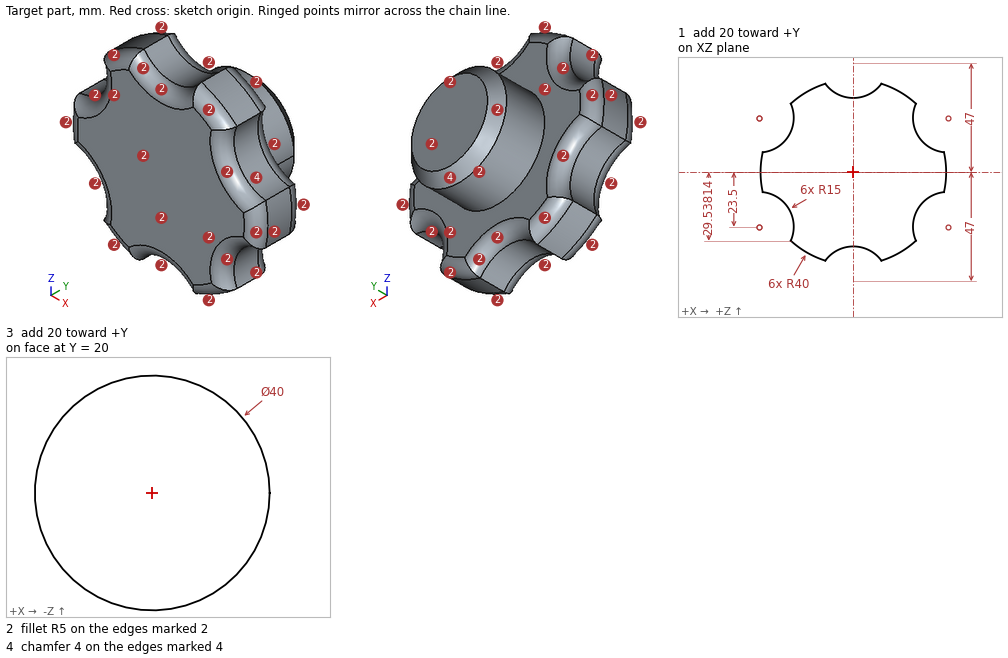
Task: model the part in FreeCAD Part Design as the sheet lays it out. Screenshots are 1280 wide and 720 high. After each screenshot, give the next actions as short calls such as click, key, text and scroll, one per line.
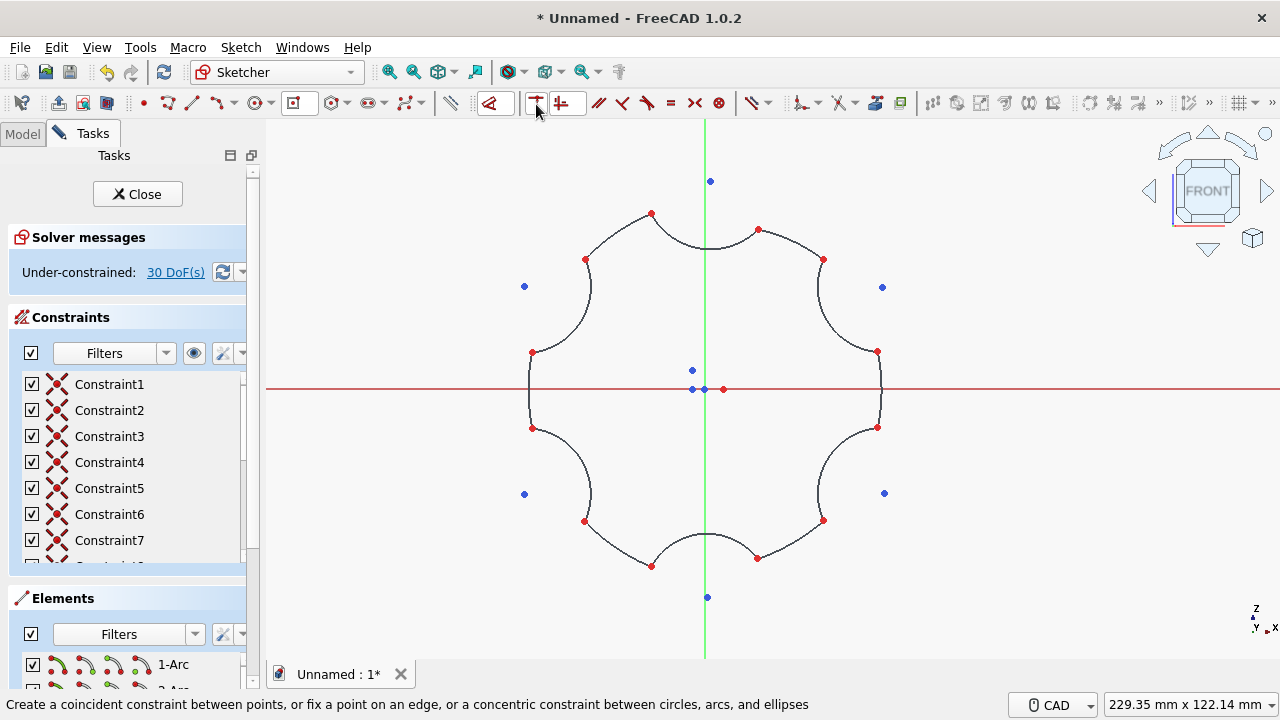
click(603, 538)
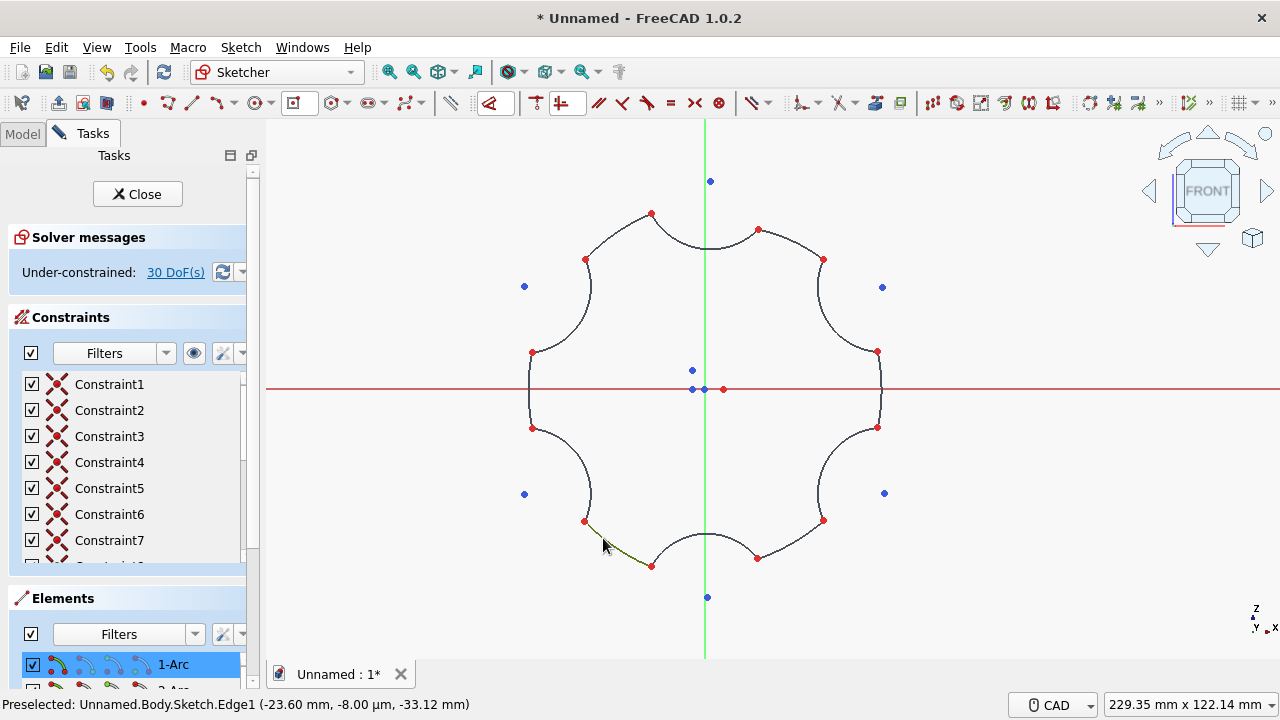
click(881, 405)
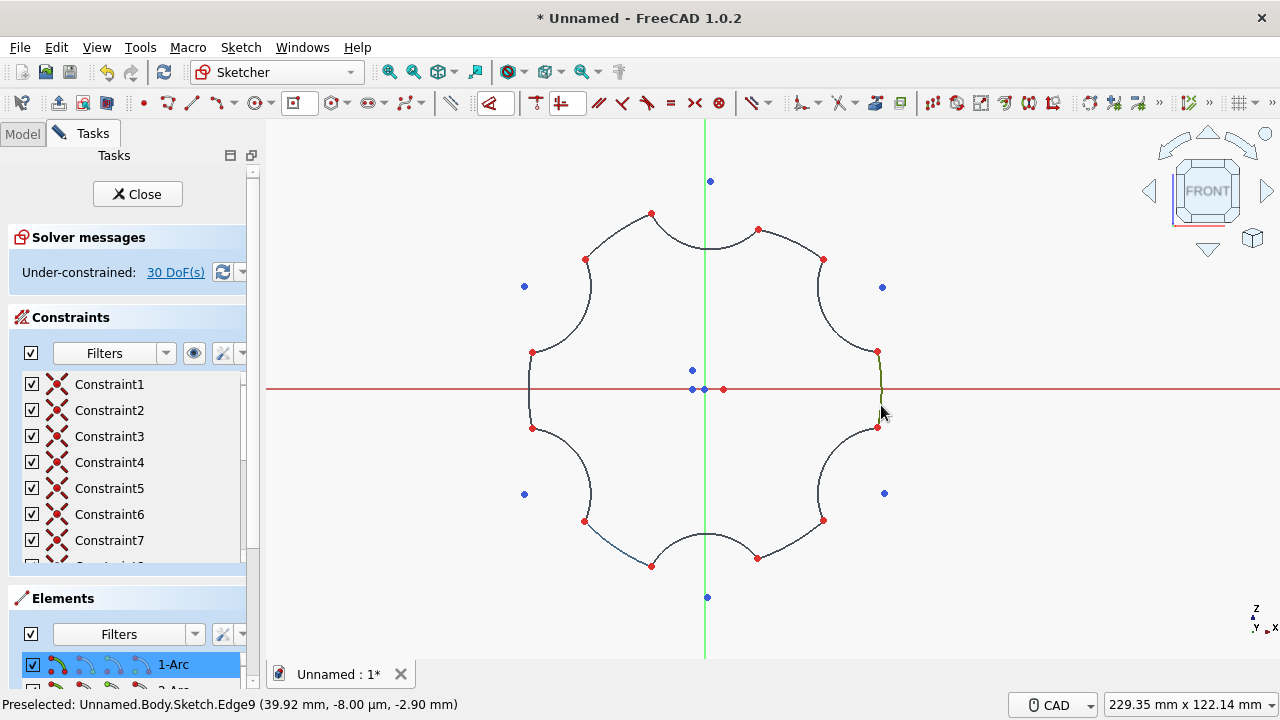
click(536, 104)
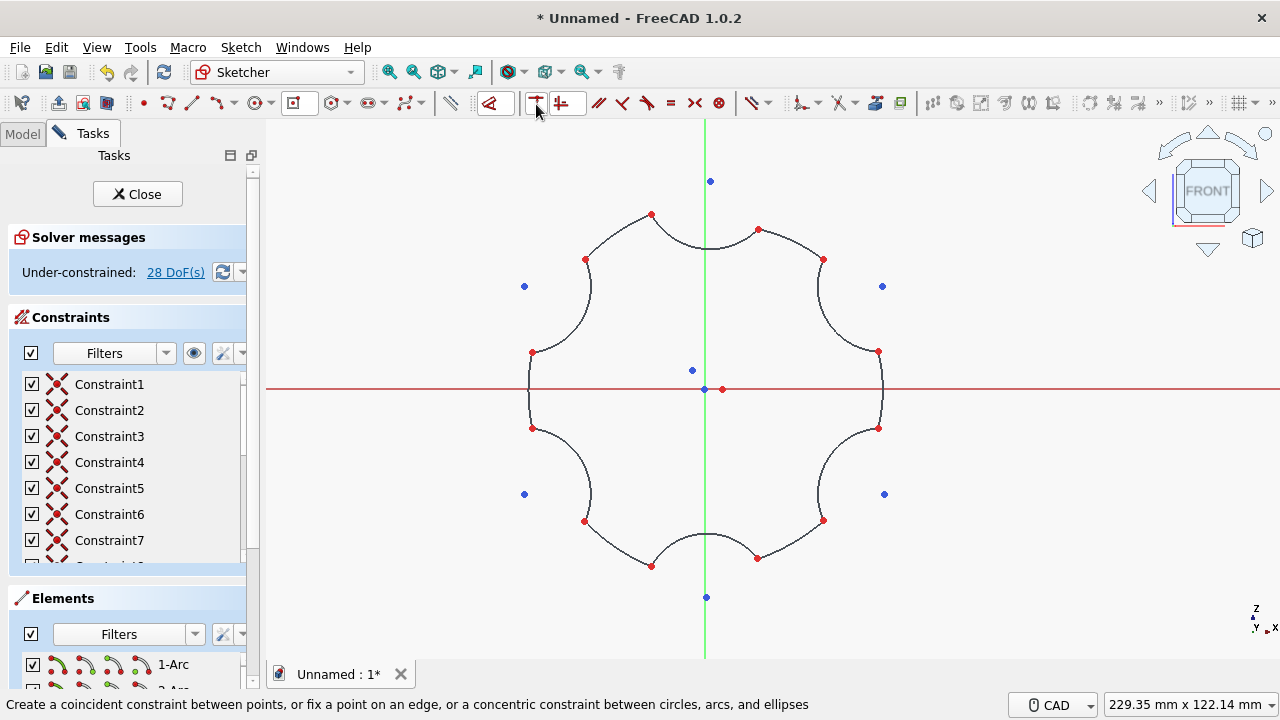
click(603, 538)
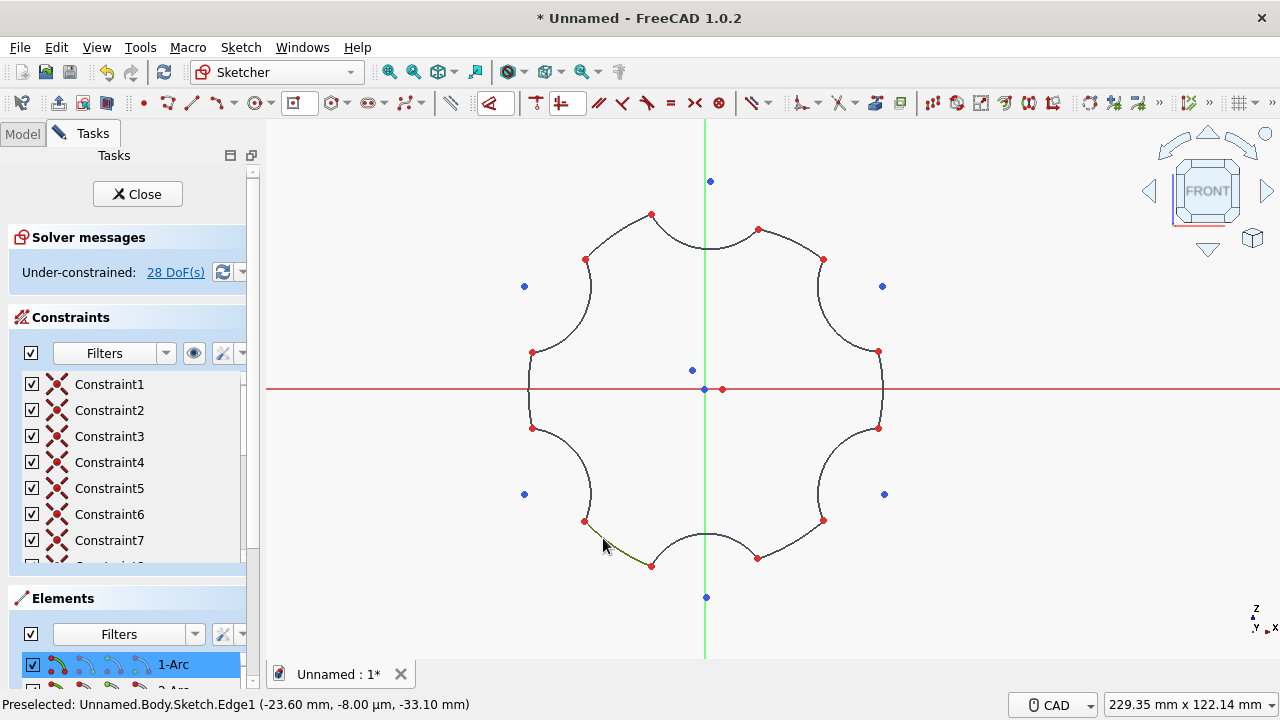
click(779, 550)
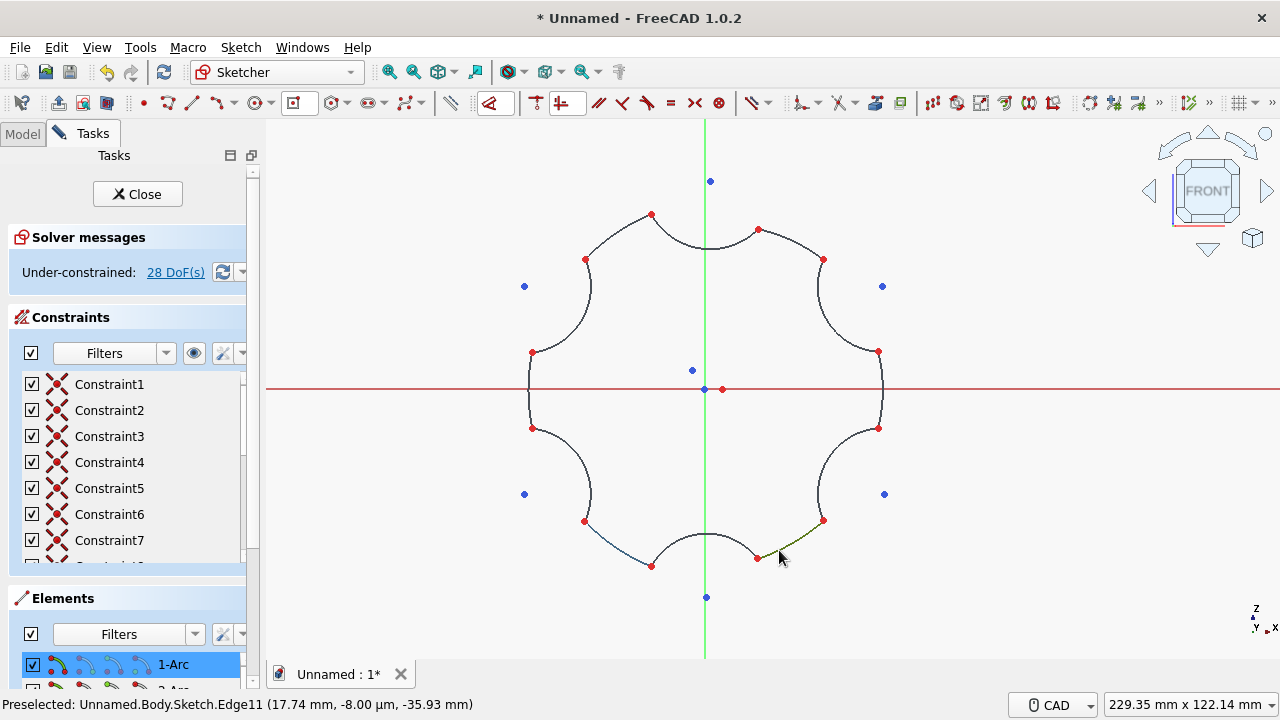
click(536, 104)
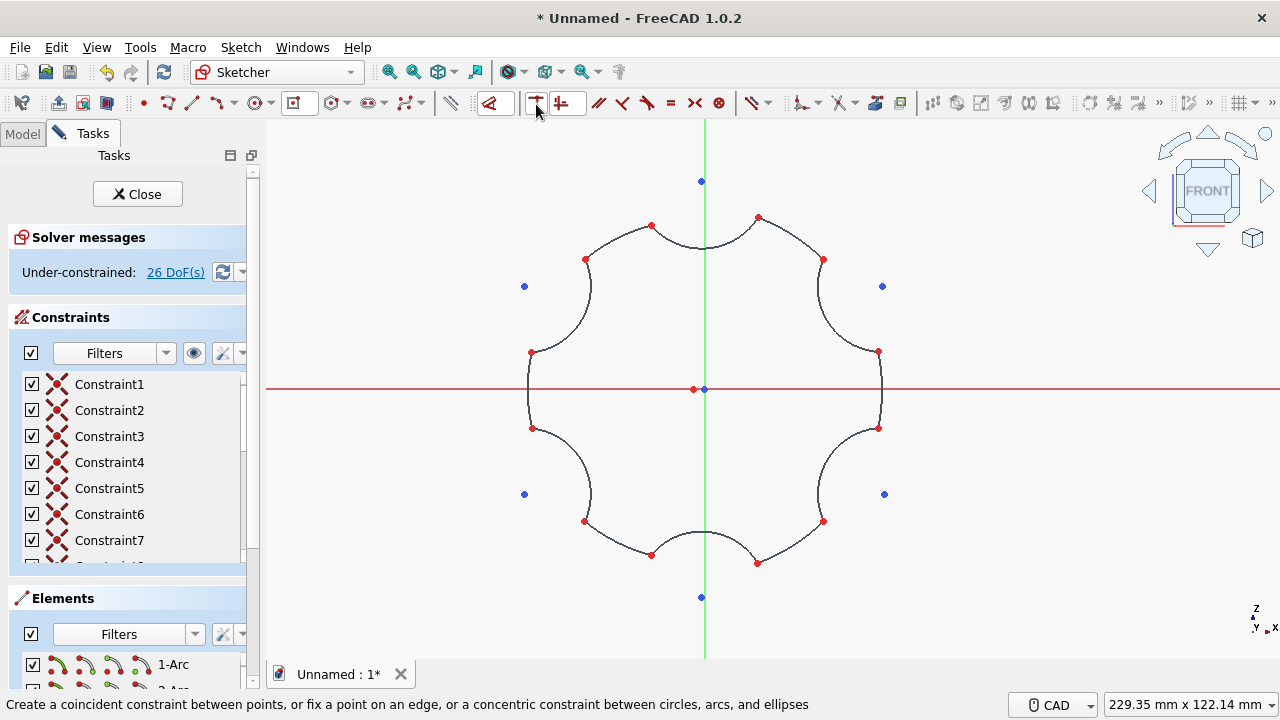
drag(683, 379, 715, 400)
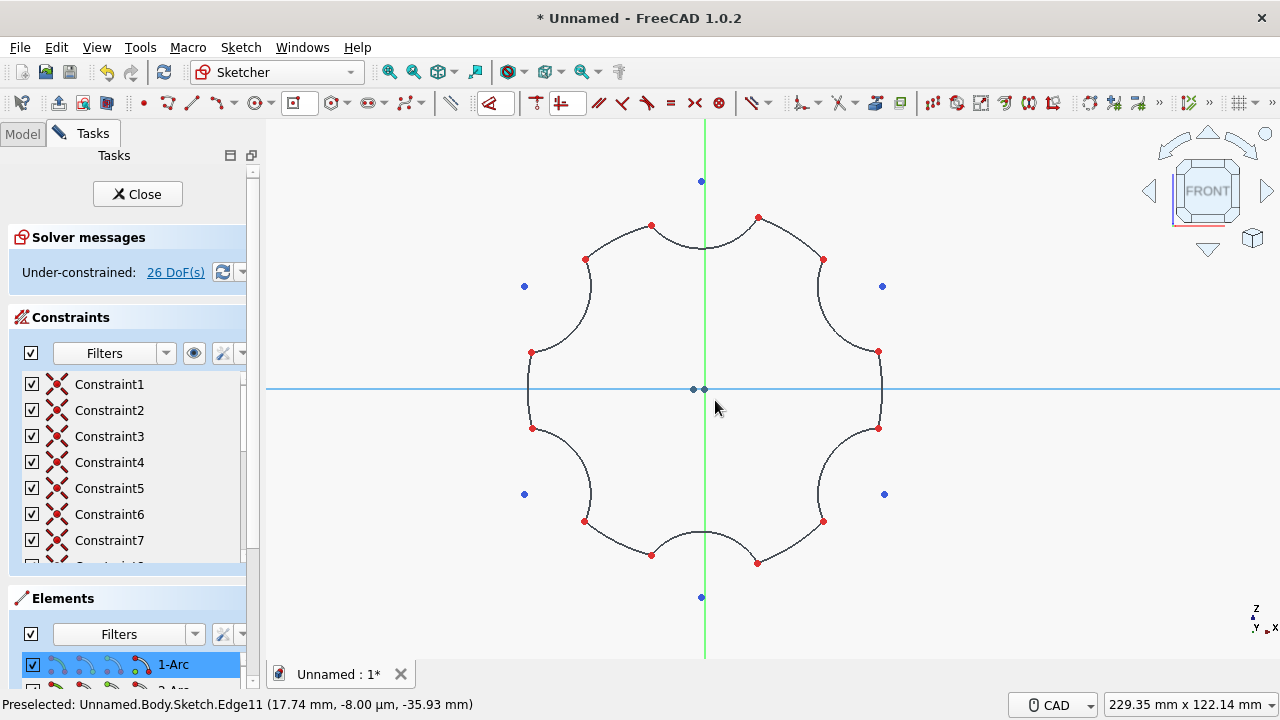
click(536, 104)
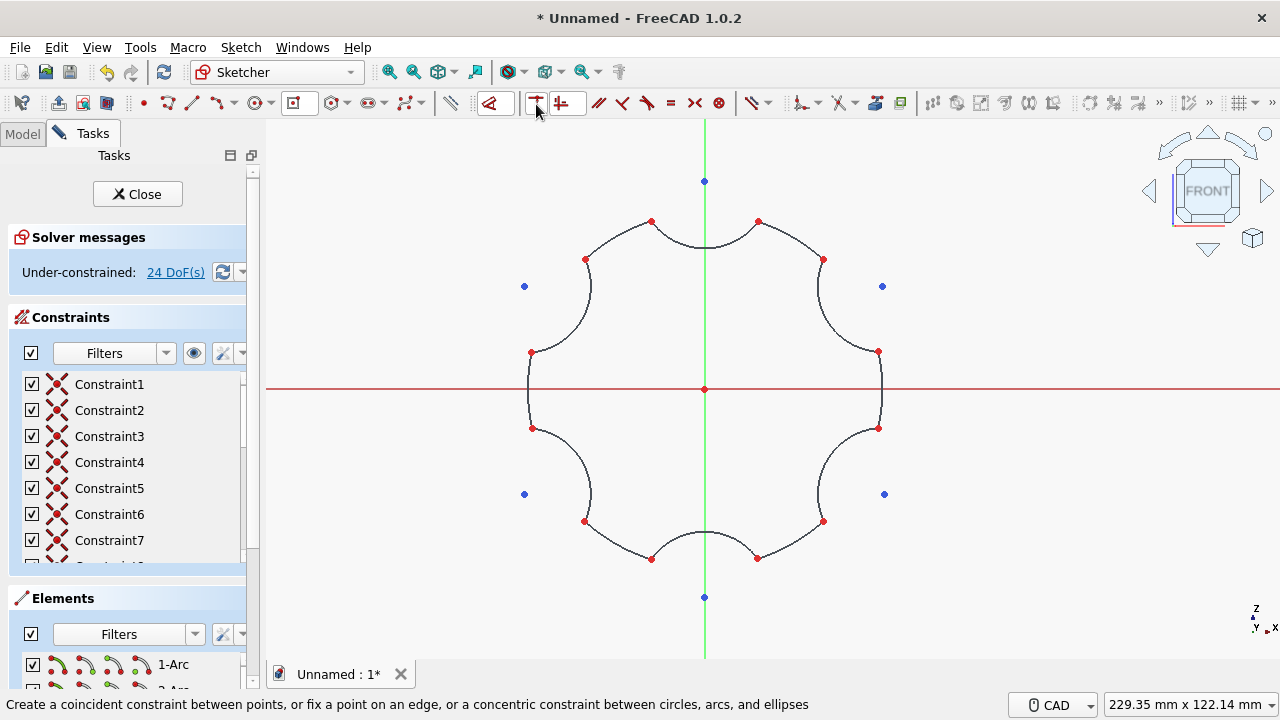
click(603, 536)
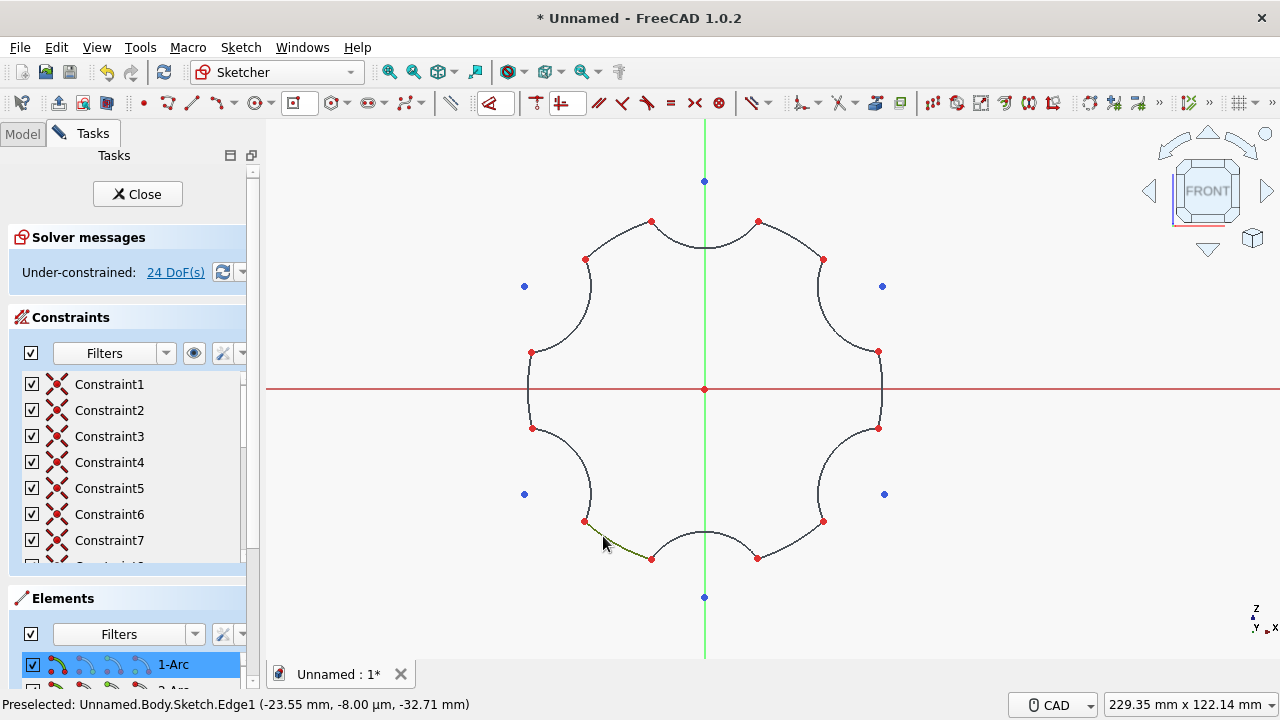
click(528, 375)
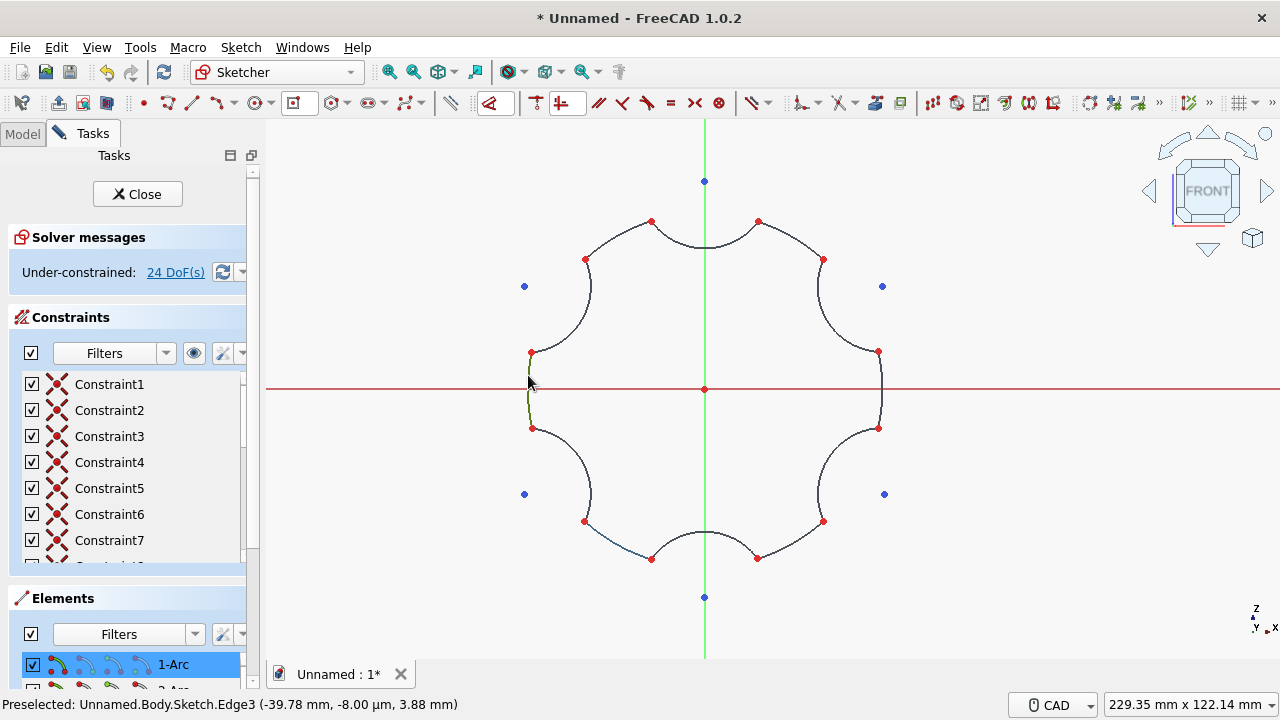
click(630, 230)